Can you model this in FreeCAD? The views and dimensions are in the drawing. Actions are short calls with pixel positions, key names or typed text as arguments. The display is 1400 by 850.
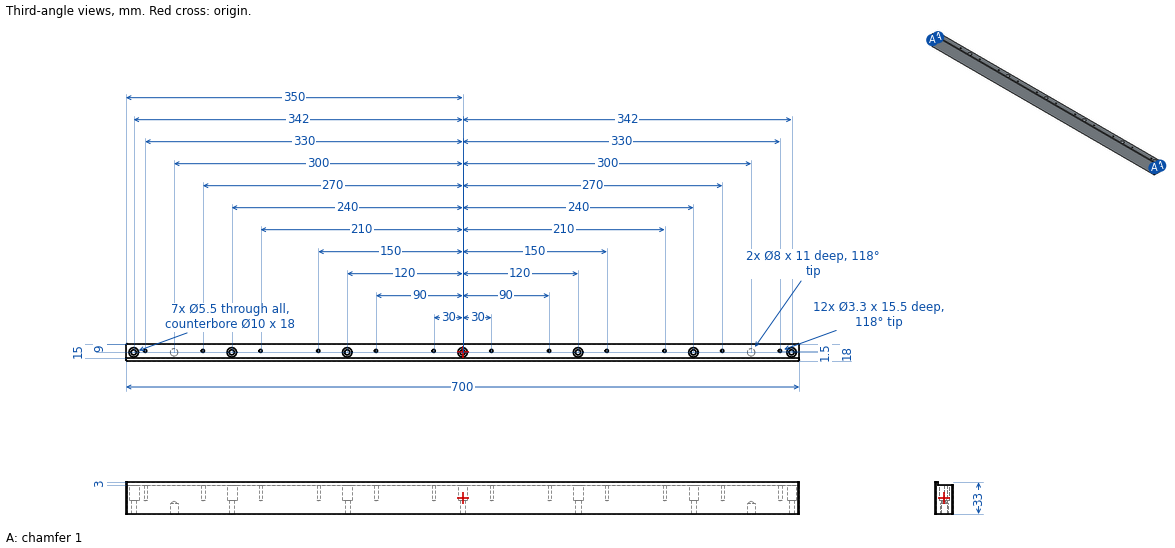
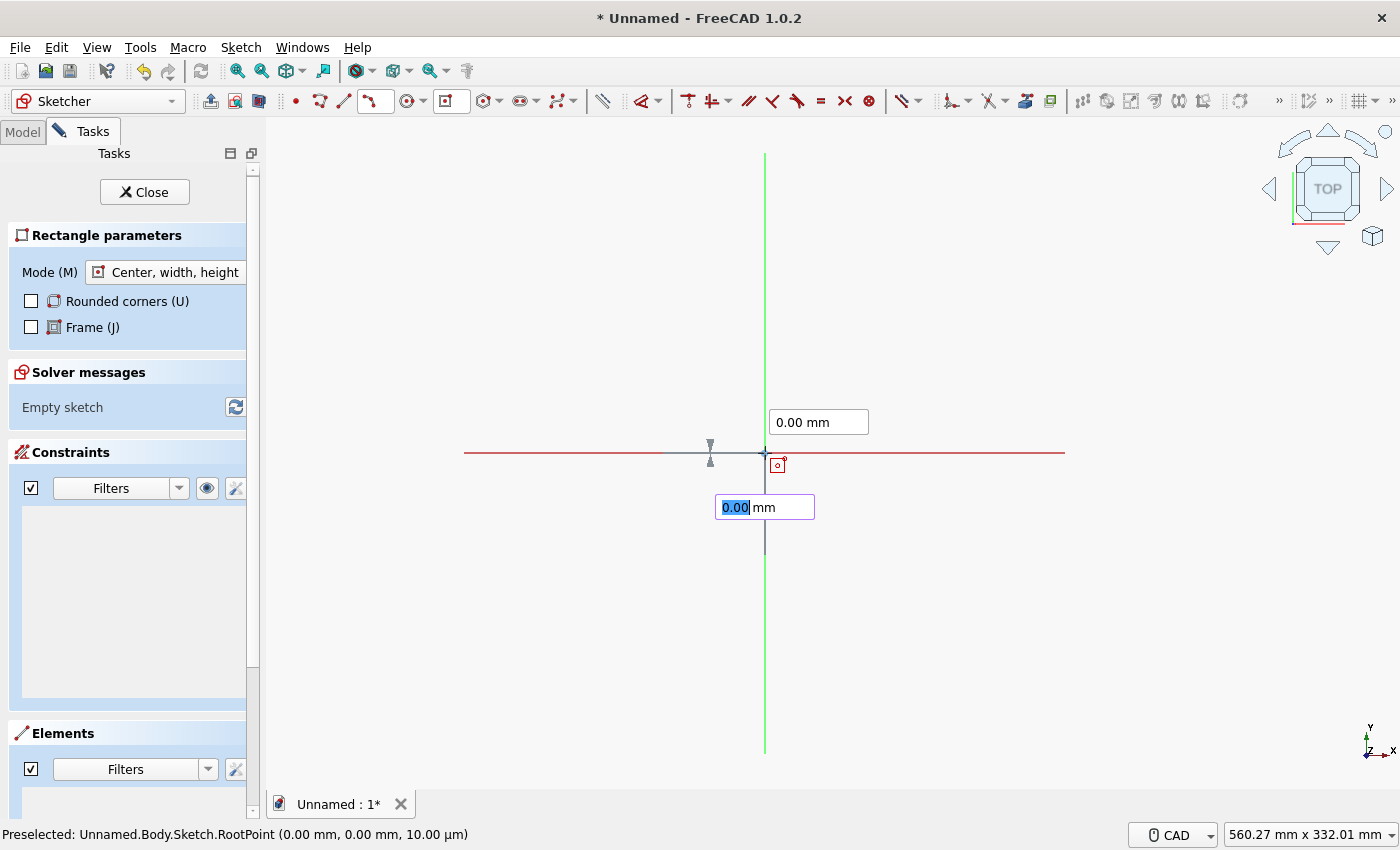
scroll(764, 453, down, 4)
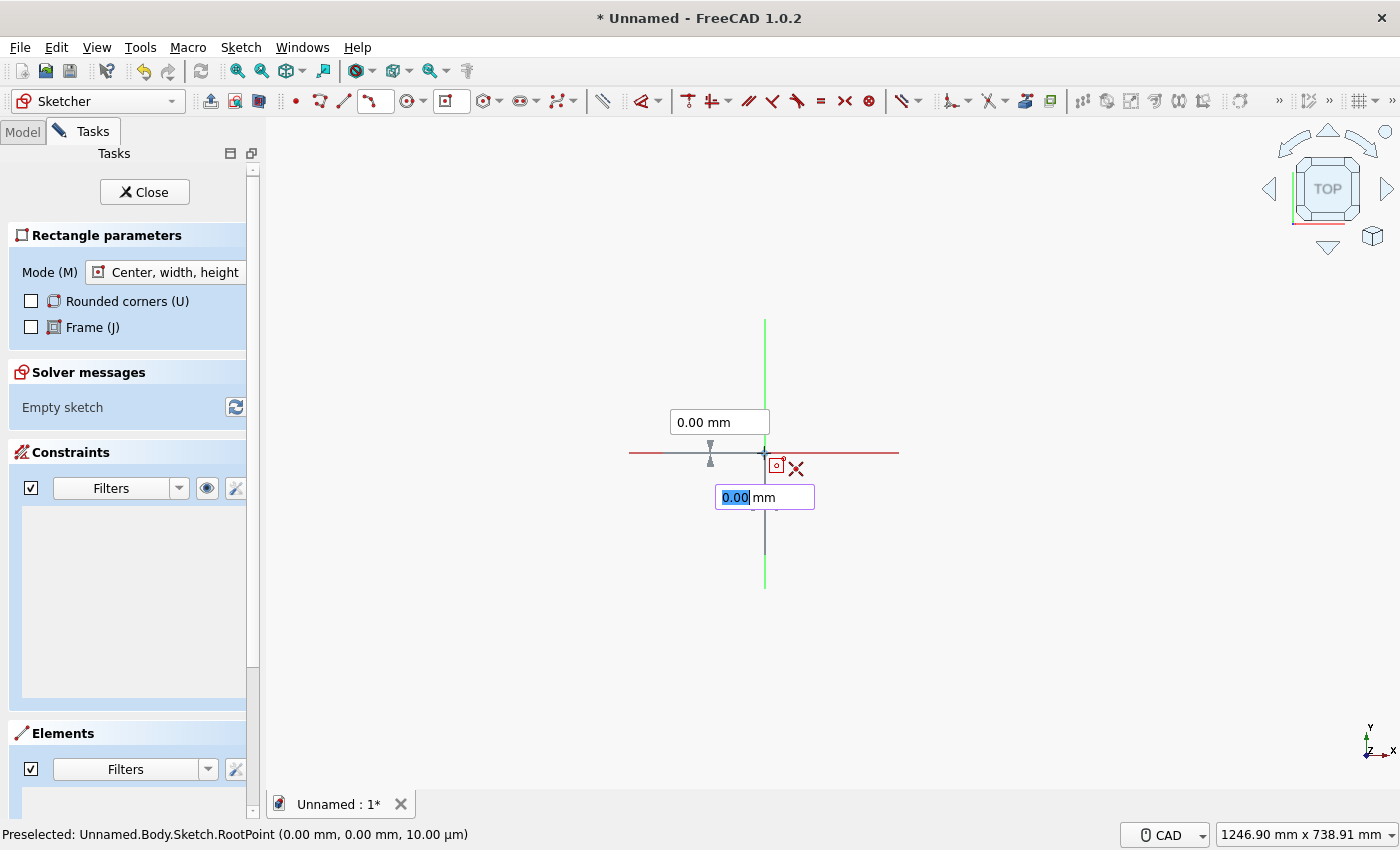
scroll(1083, 445, up, 4)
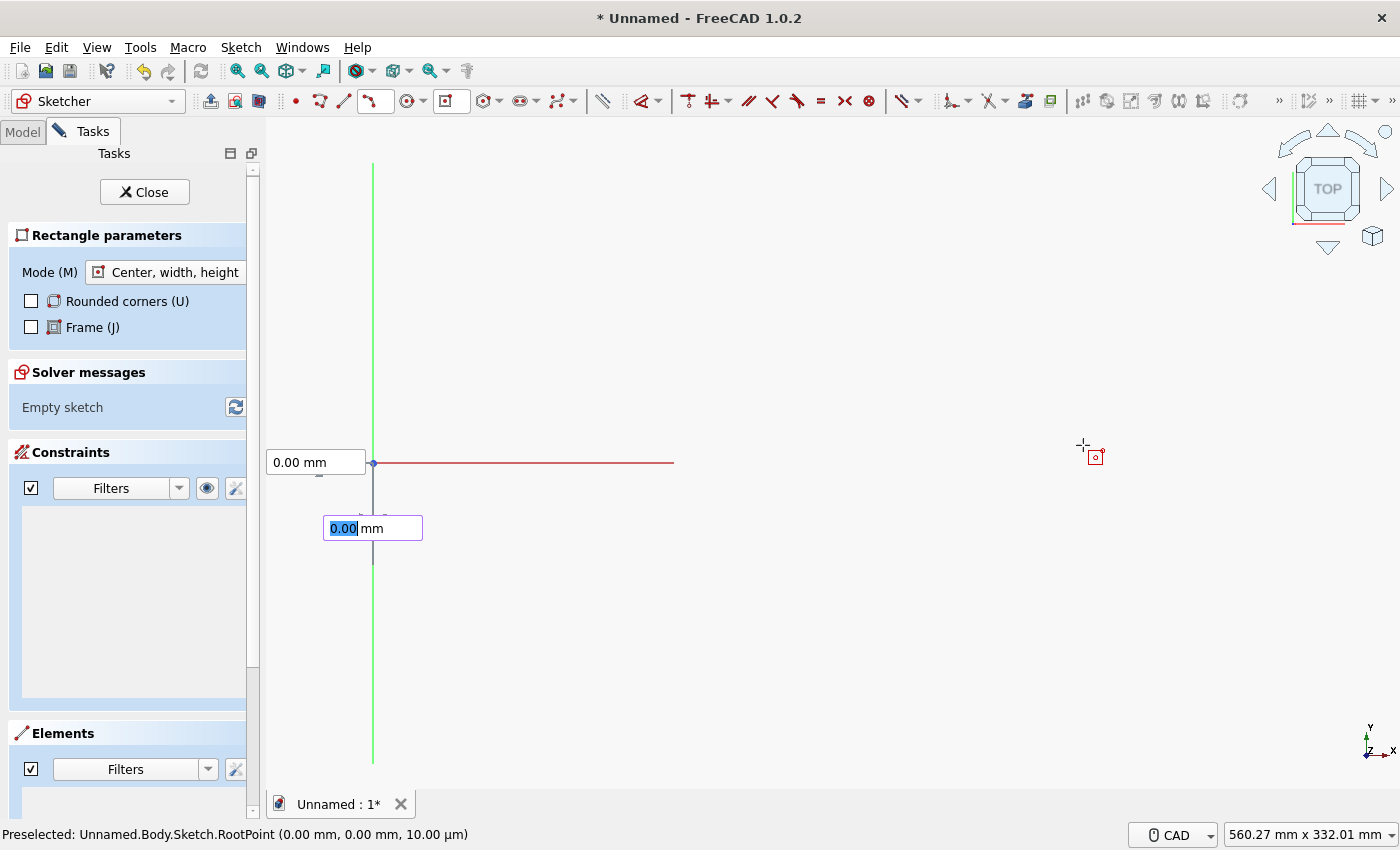
click(1082, 445)
key(Escape)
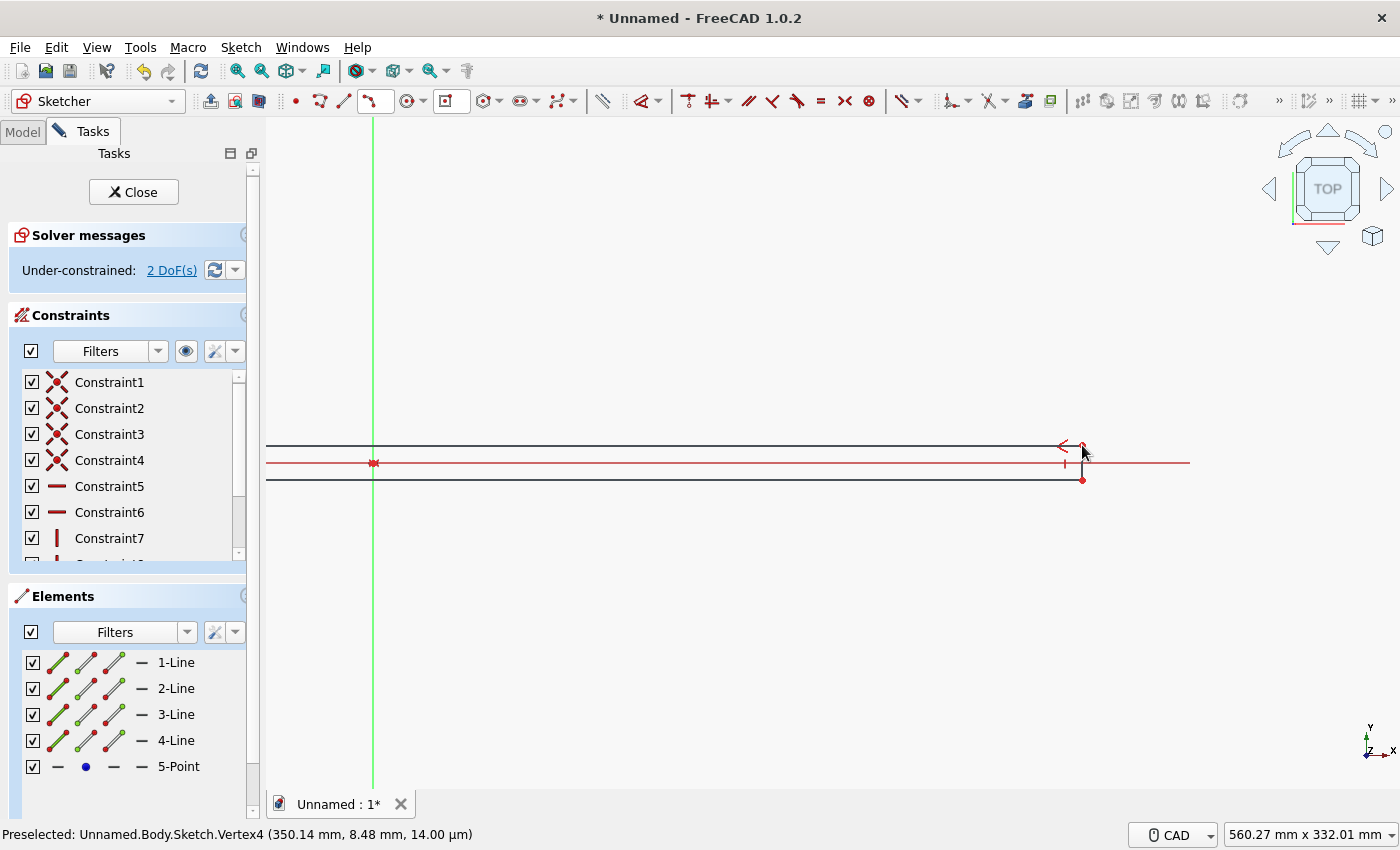
key(d)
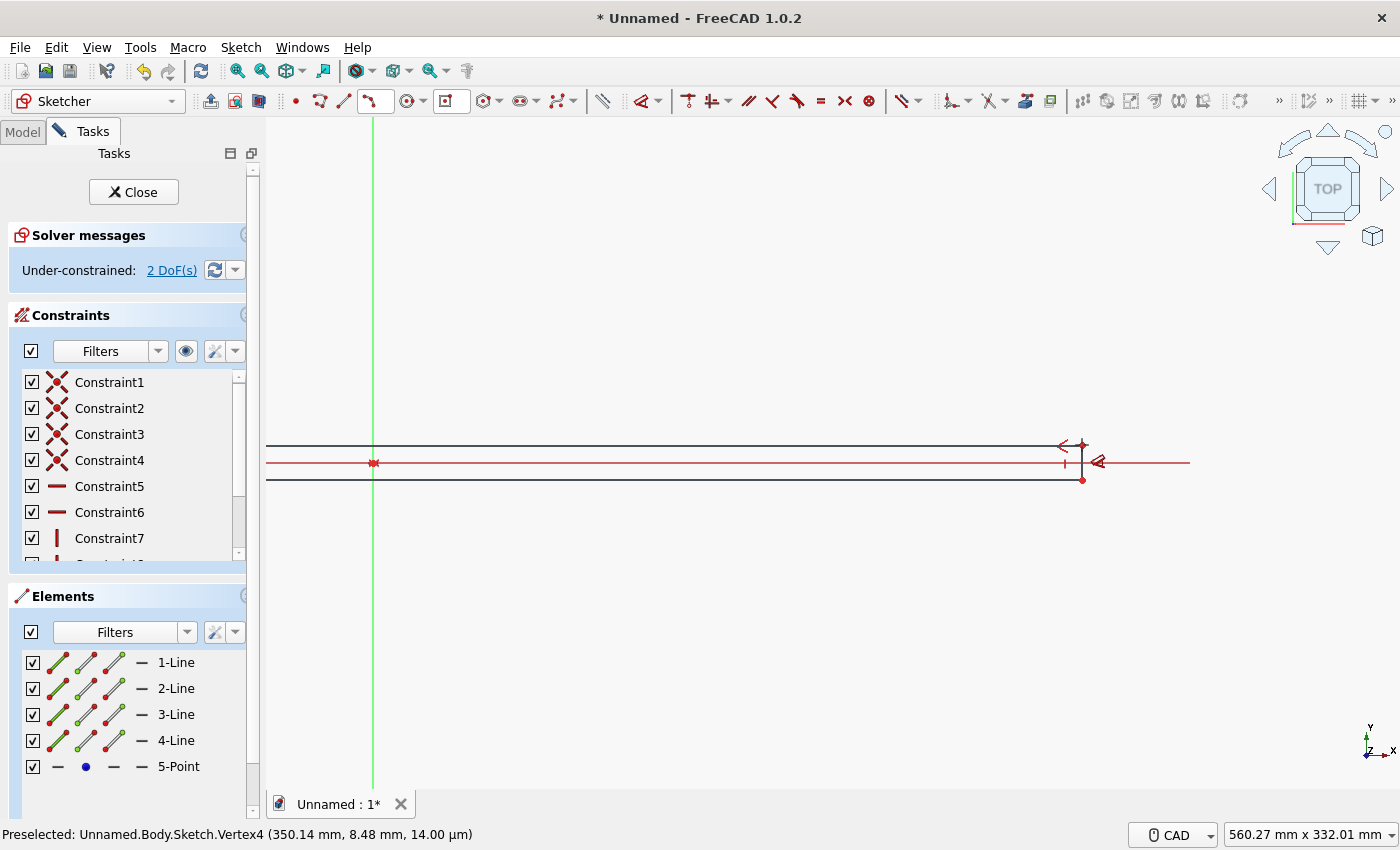
click(1082, 467)
click(1116, 455)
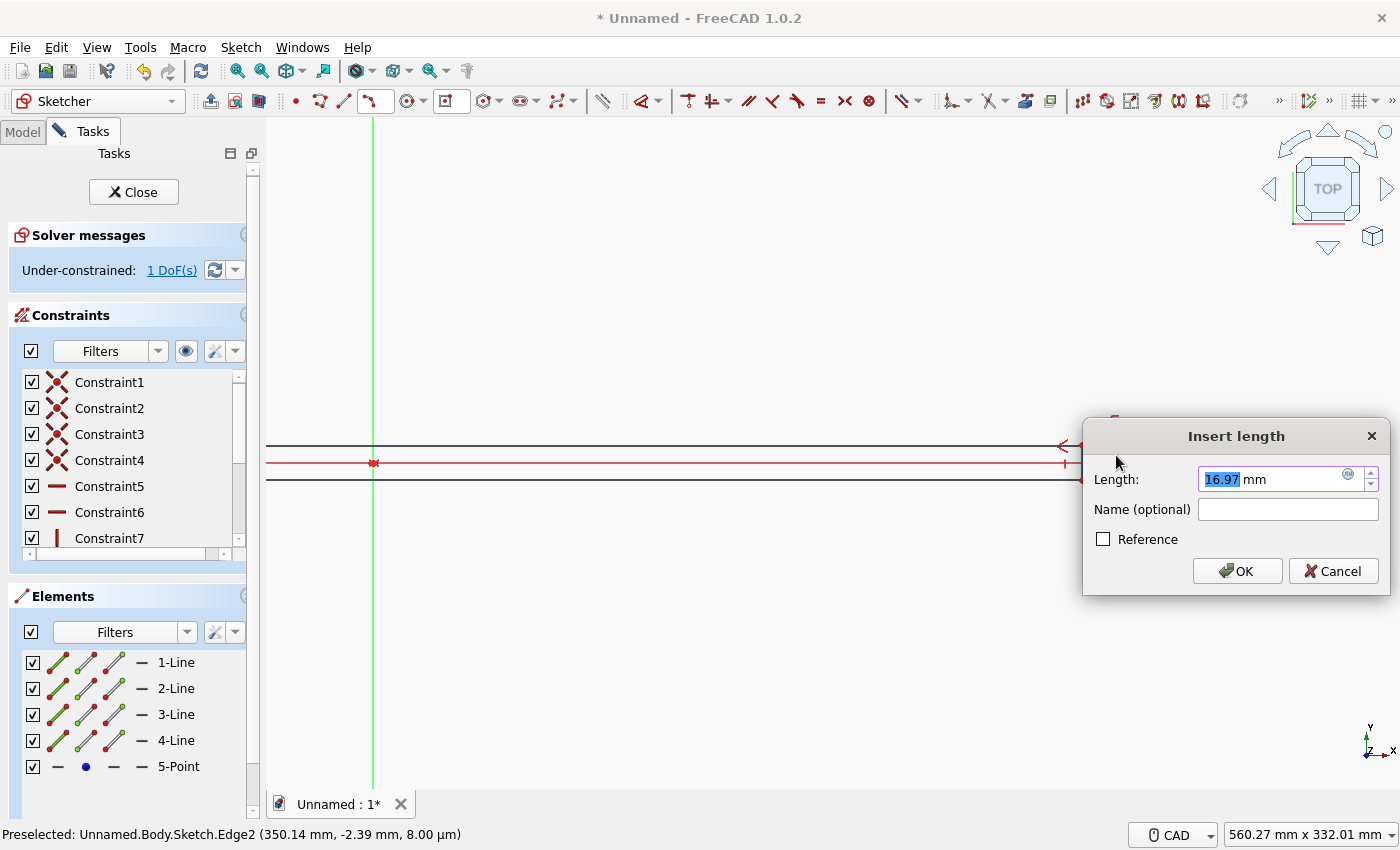
text(18)
key(Return)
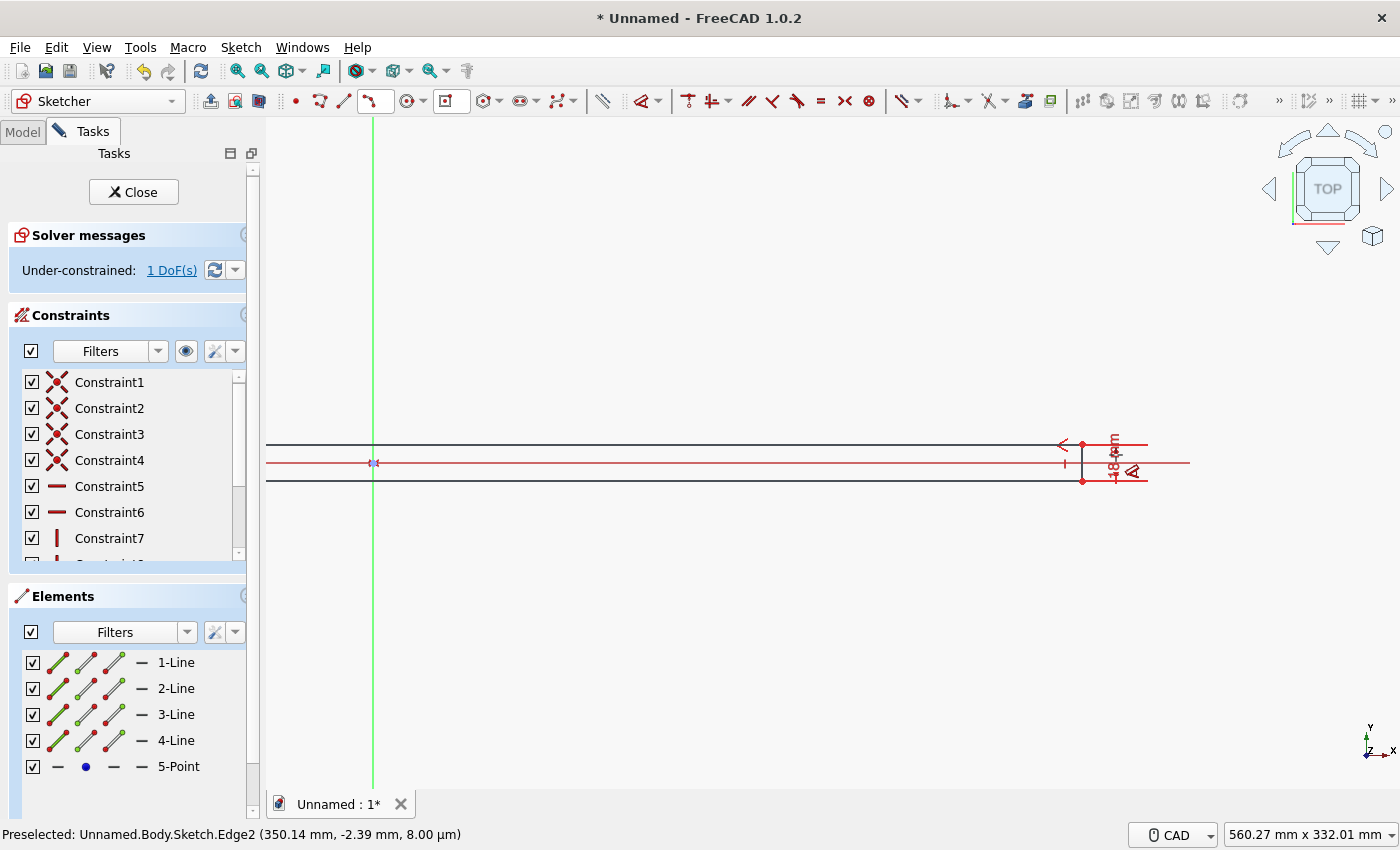
click(657, 481)
click(688, 515)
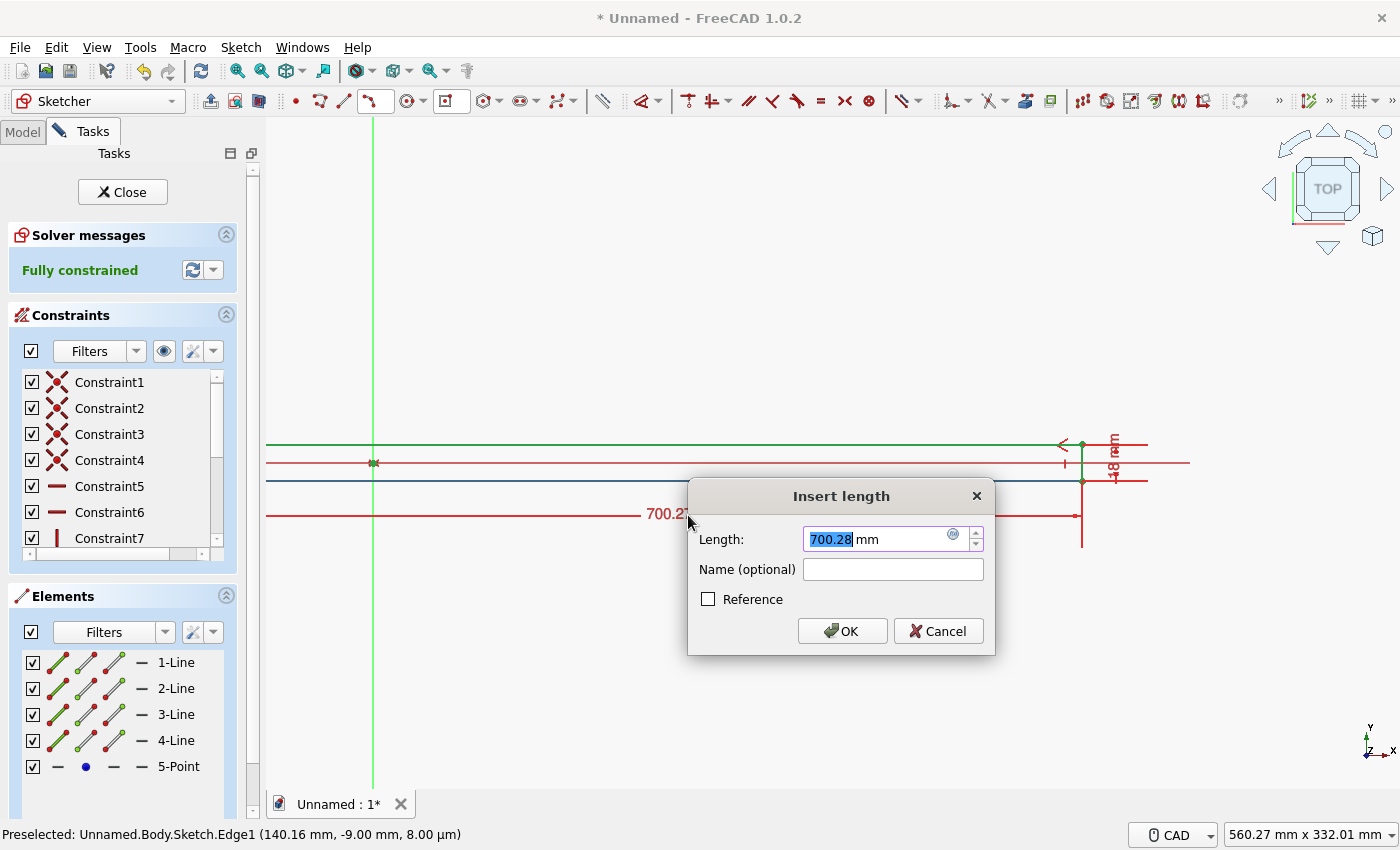
text(700)
key(Return)
key(Escape)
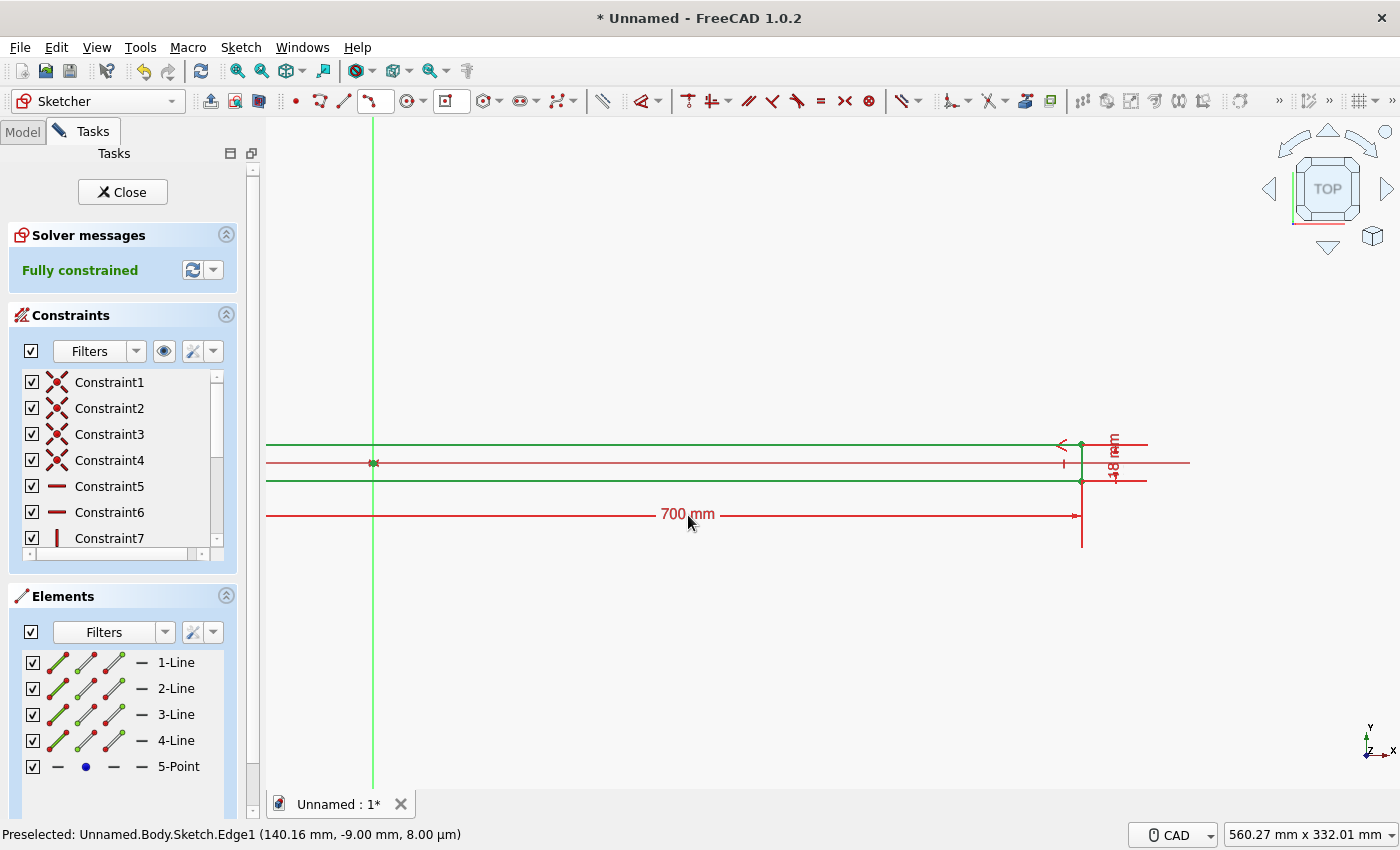
click(123, 192)